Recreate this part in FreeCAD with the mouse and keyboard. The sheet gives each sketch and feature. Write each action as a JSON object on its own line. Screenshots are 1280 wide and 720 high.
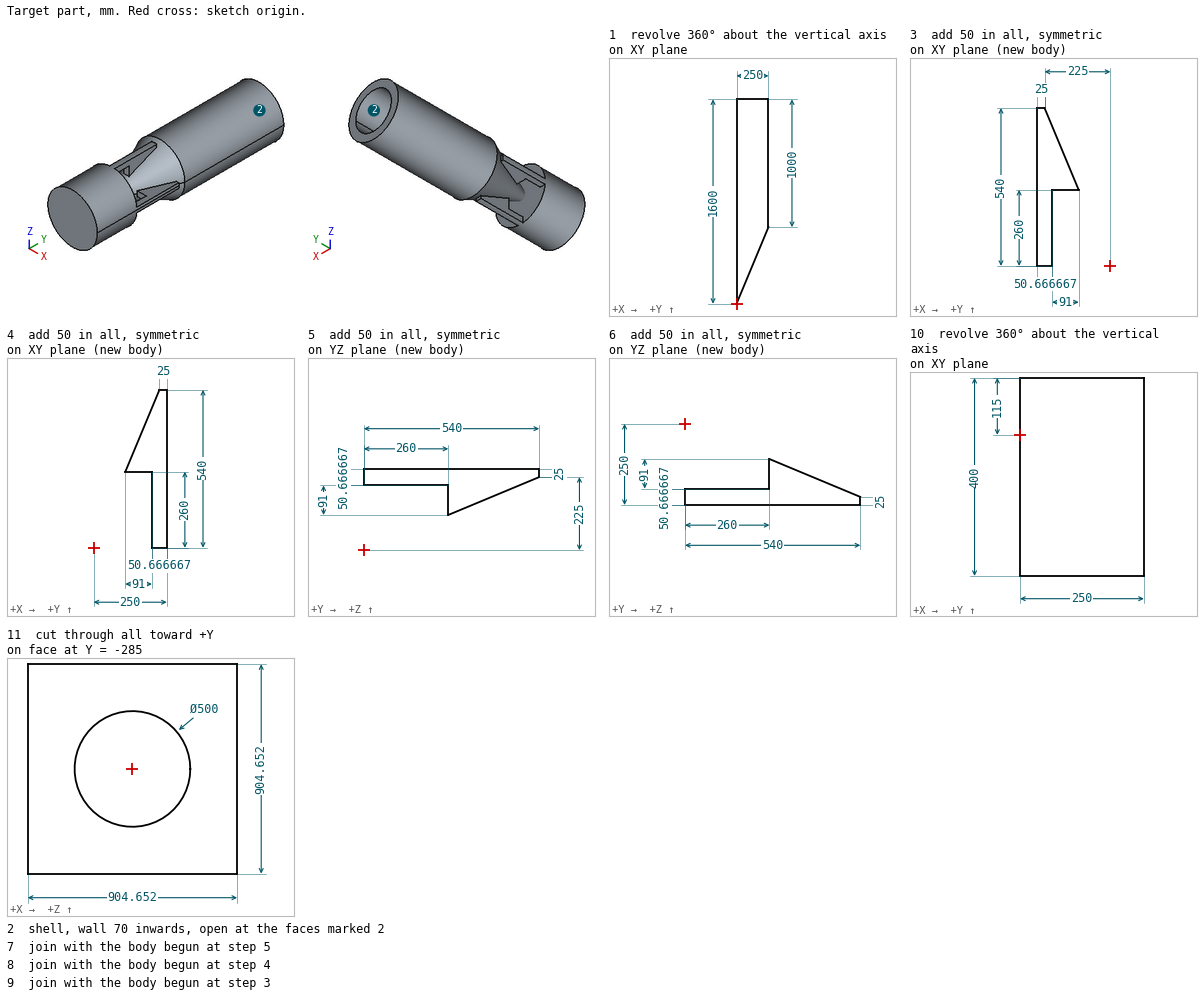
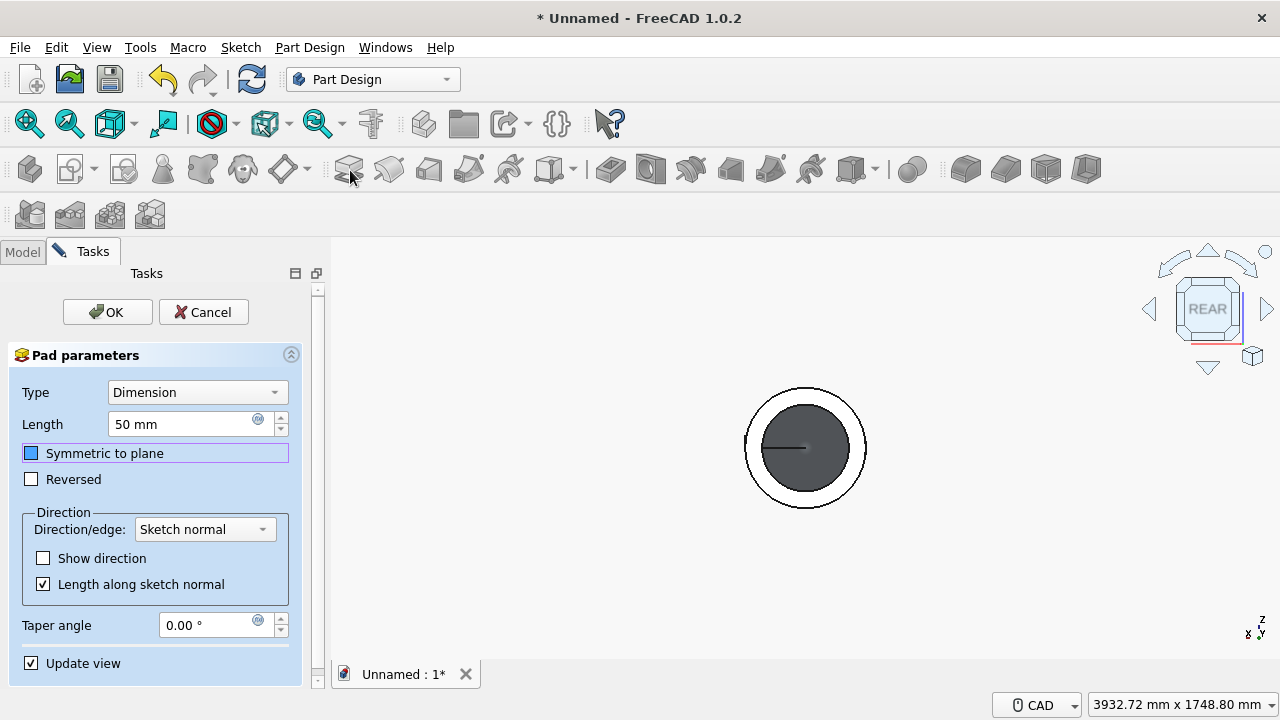
{"action": "left_click", "coordinate": [30, 453]}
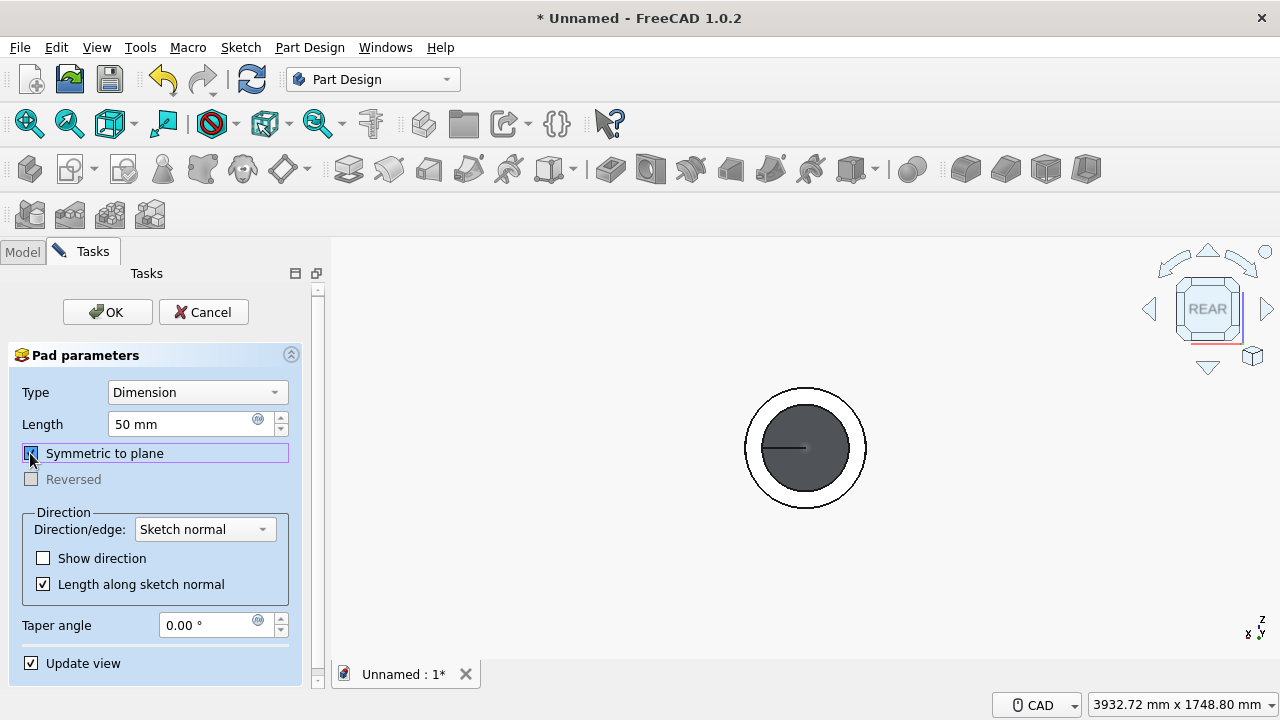
{"action": "left_click", "coordinate": [108, 312]}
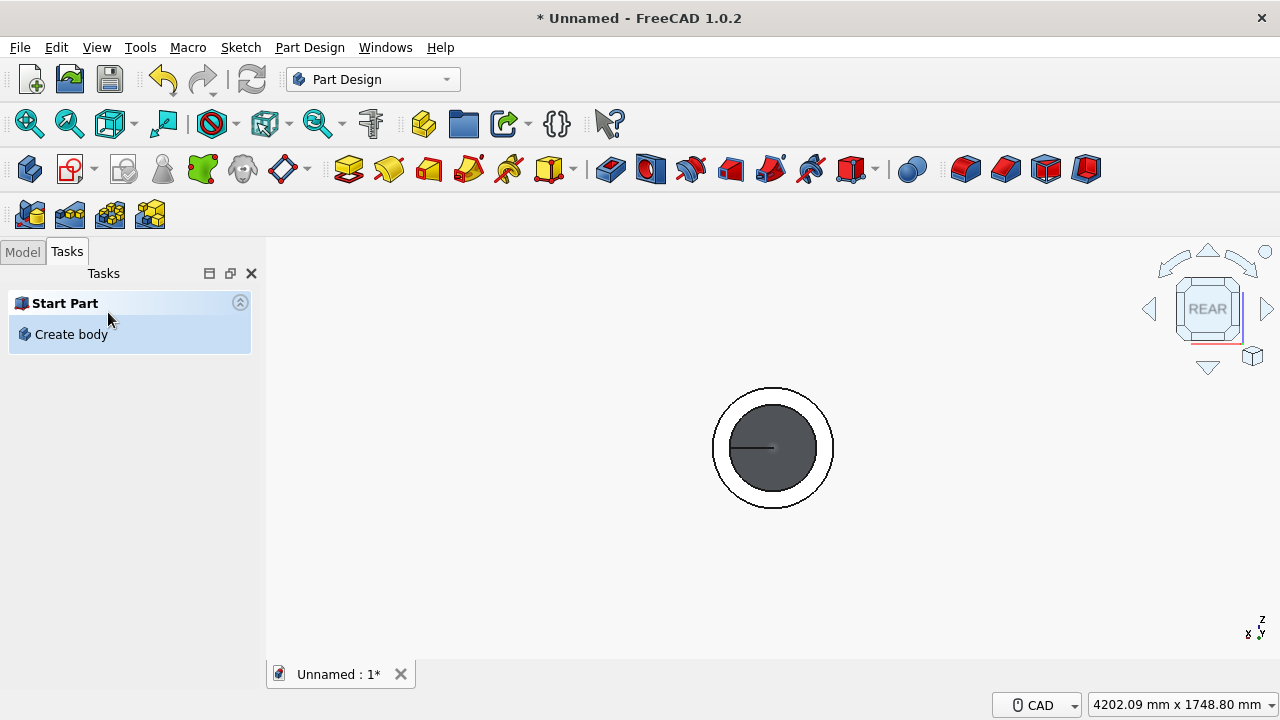
{"action": "left_click", "coordinate": [30, 124]}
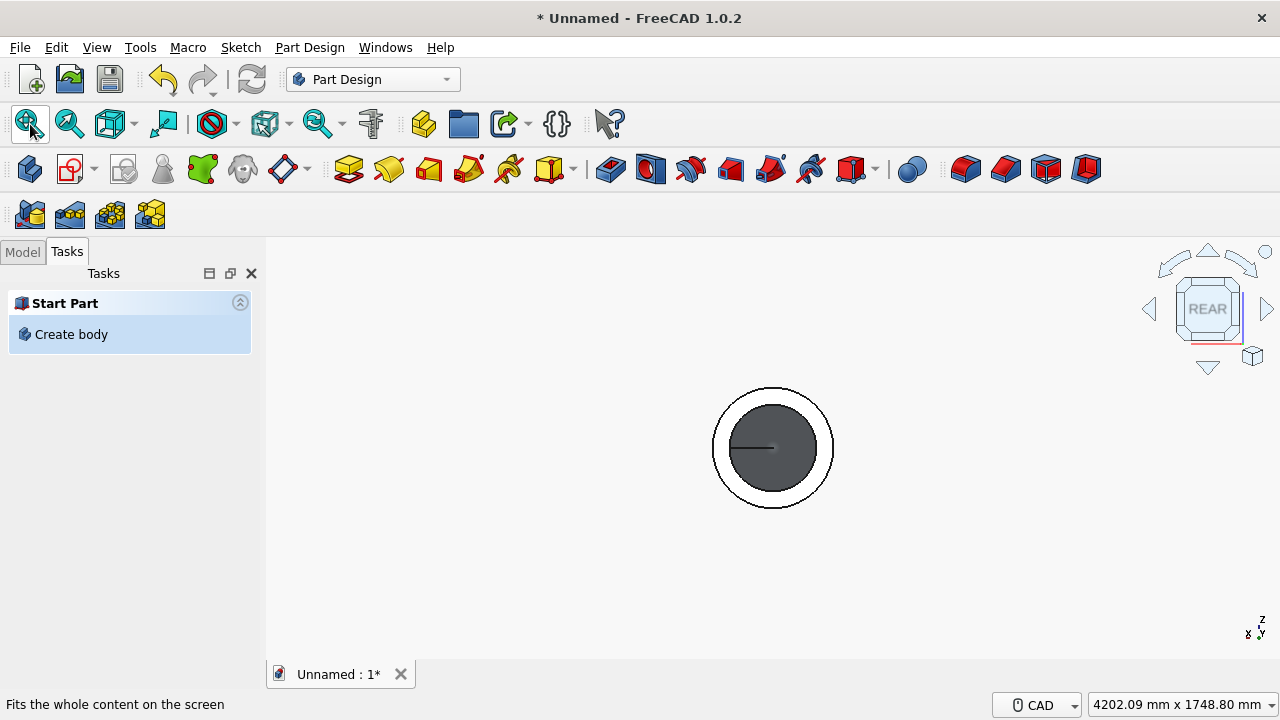
{"action": "left_click", "coordinate": [30, 170]}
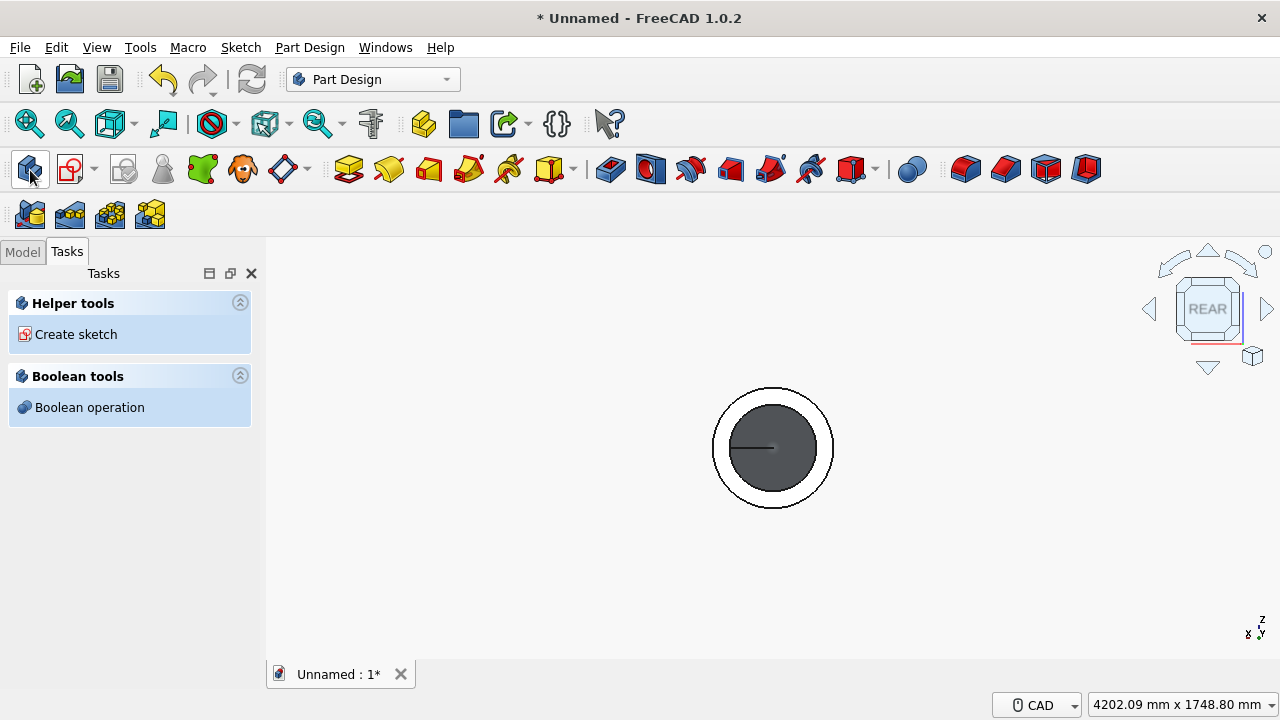
{"action": "left_click", "coordinate": [306, 619]}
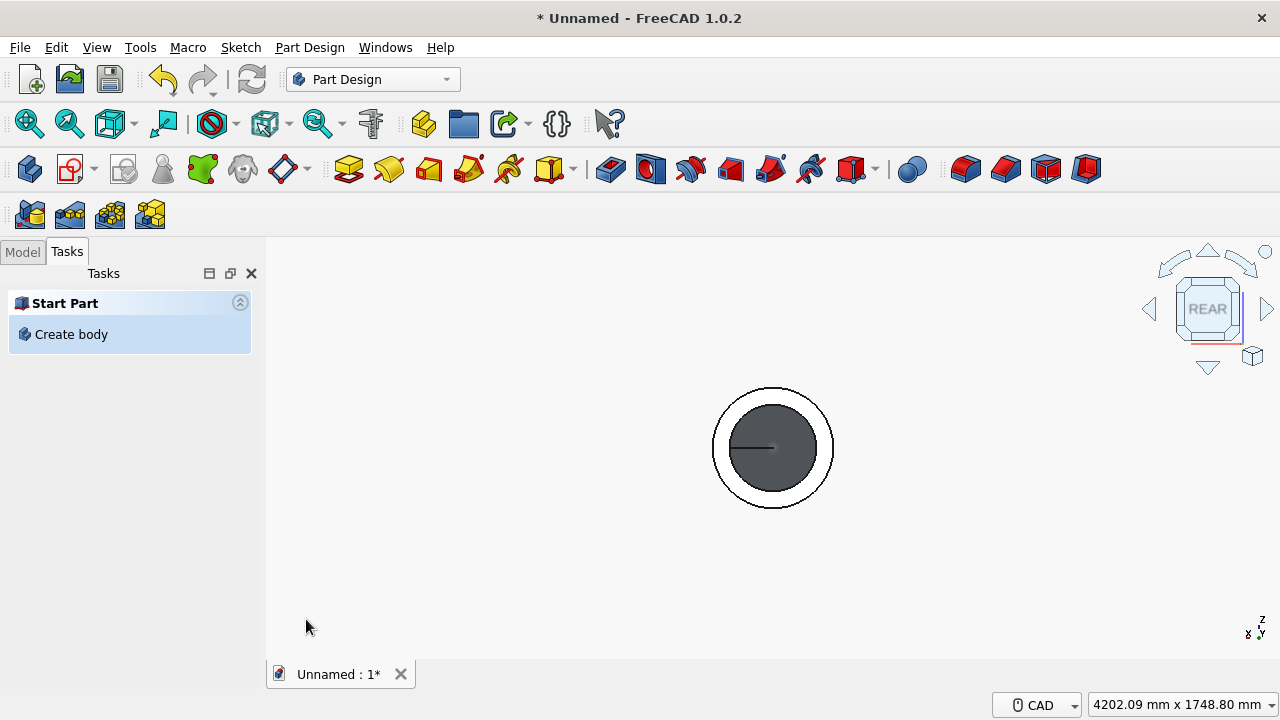
{"action": "left_click", "coordinate": [70, 170]}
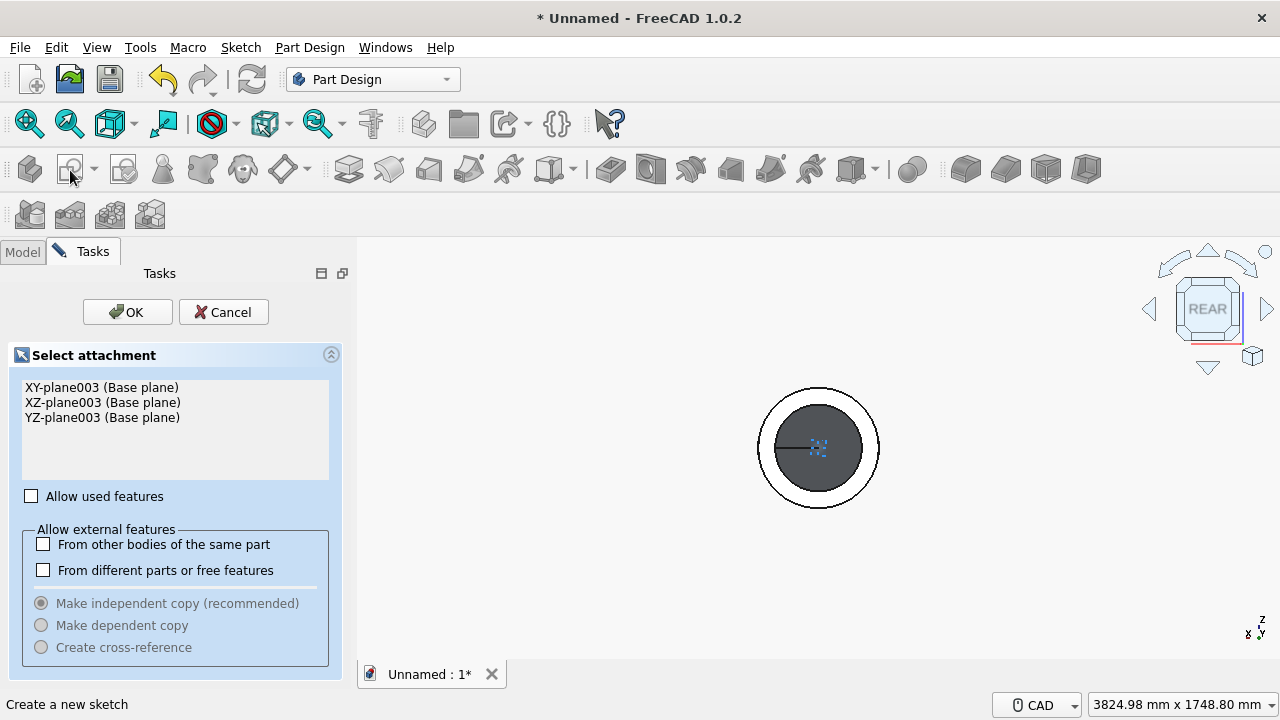
{"action": "left_click", "coordinate": [82, 418]}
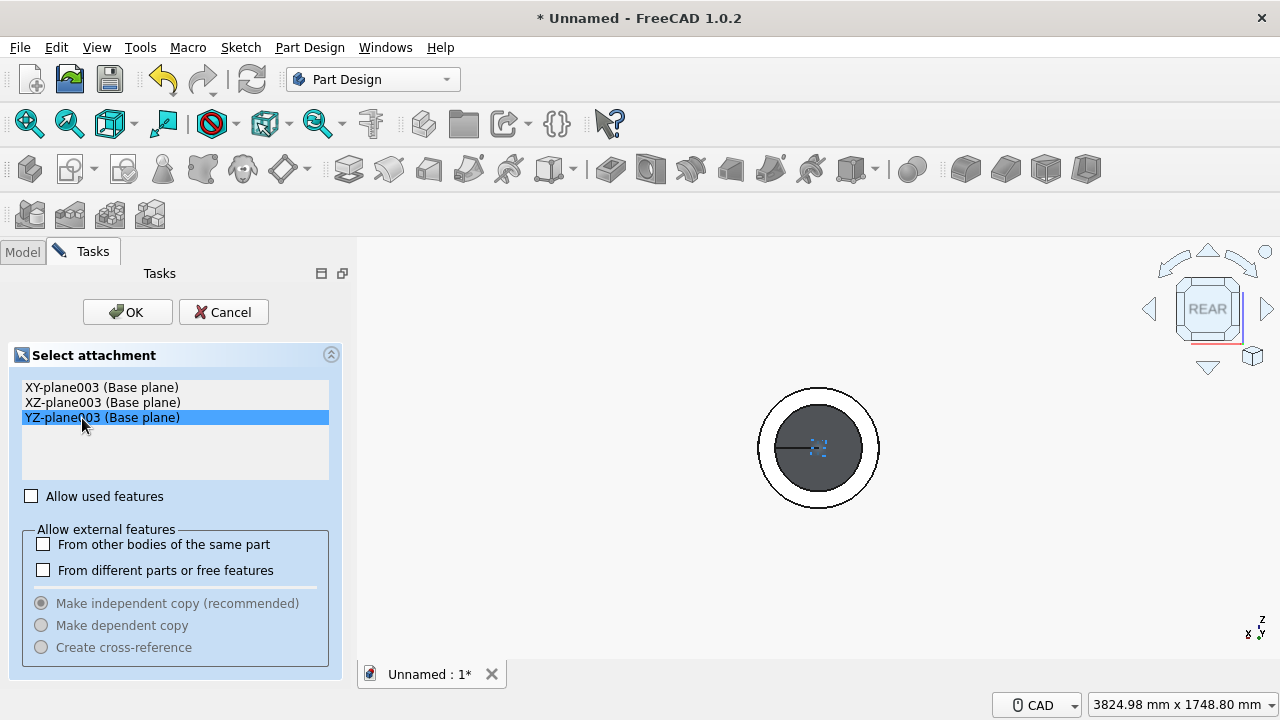
{"action": "left_click", "coordinate": [128, 312]}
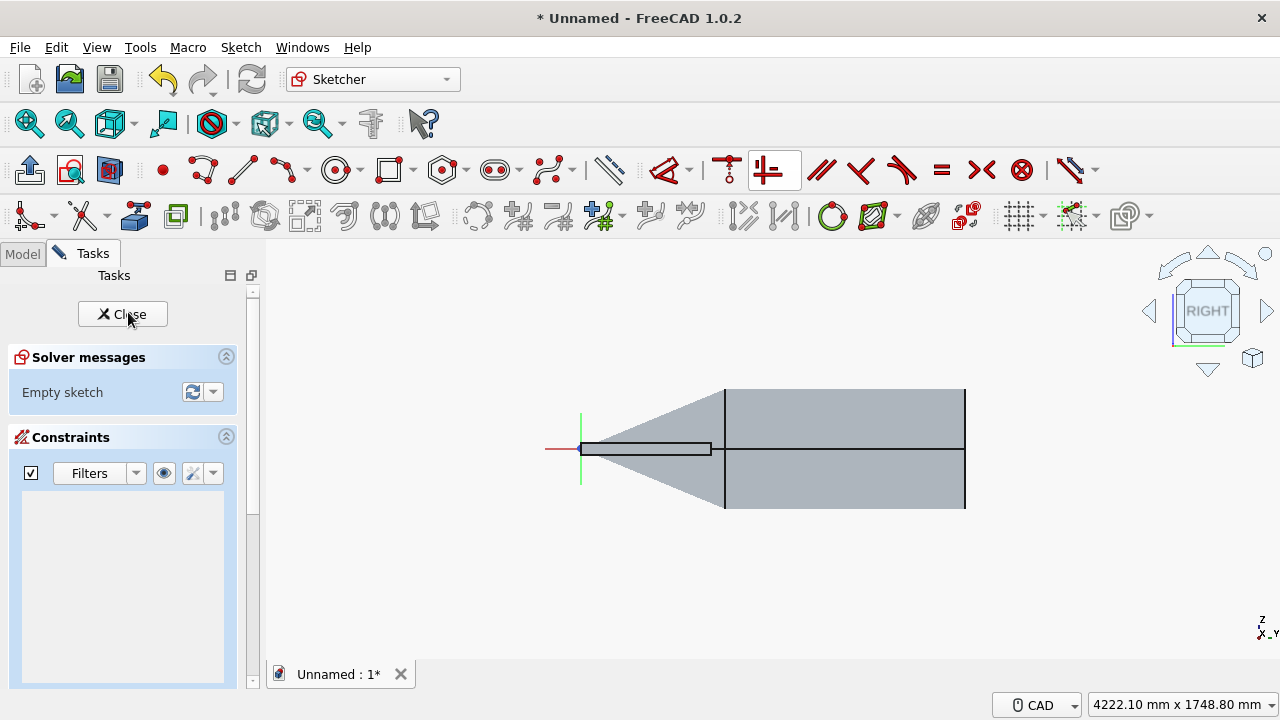
{"action": "scroll", "coordinate": [626, 409], "scroll_direction": "up", "scroll_amount": 7}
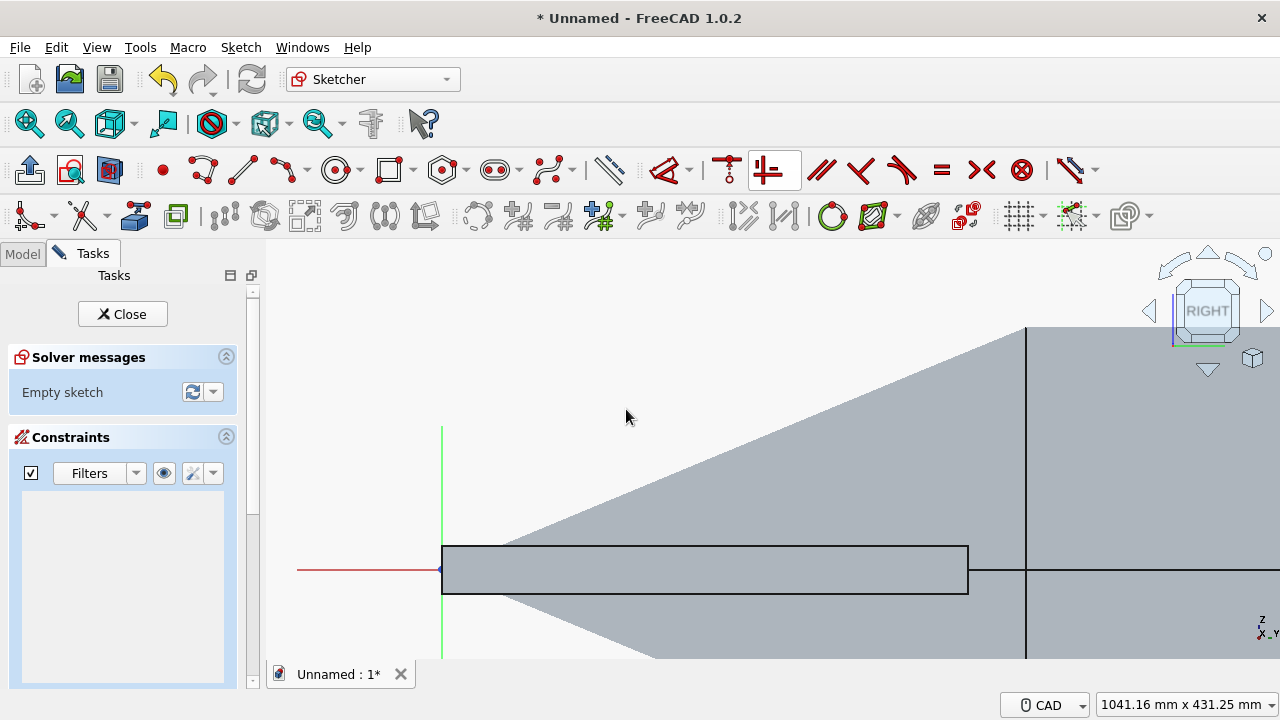
{"action": "left_click", "coordinate": [204, 170]}